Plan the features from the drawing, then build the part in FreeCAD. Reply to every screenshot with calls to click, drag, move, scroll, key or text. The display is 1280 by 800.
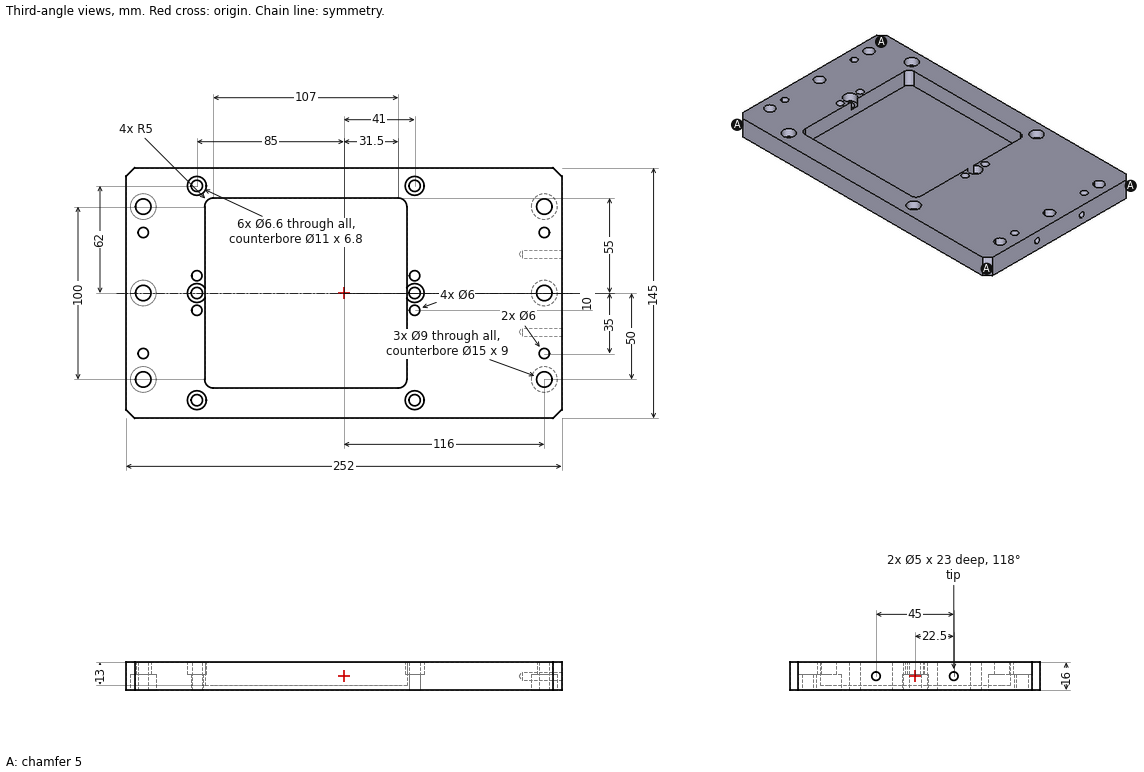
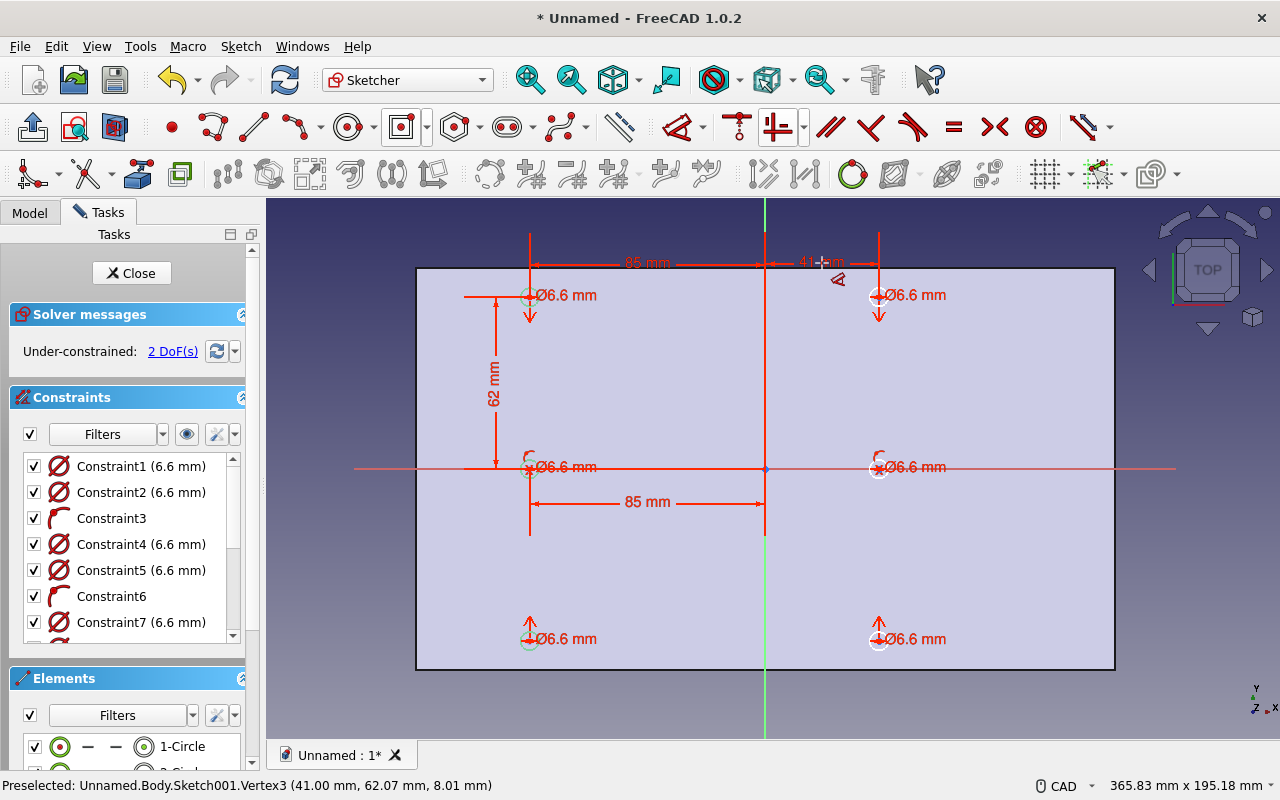
click(879, 297)
click(913, 383)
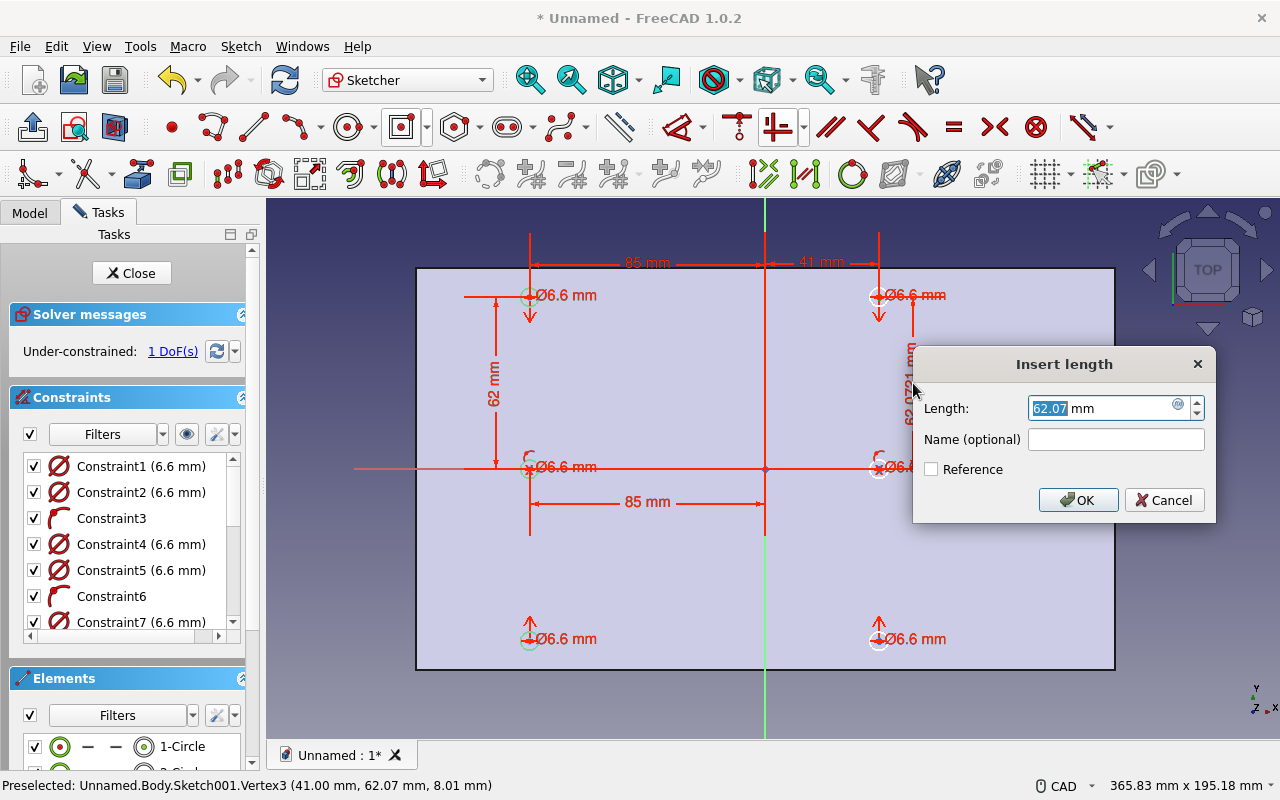
text(62)
key(Return)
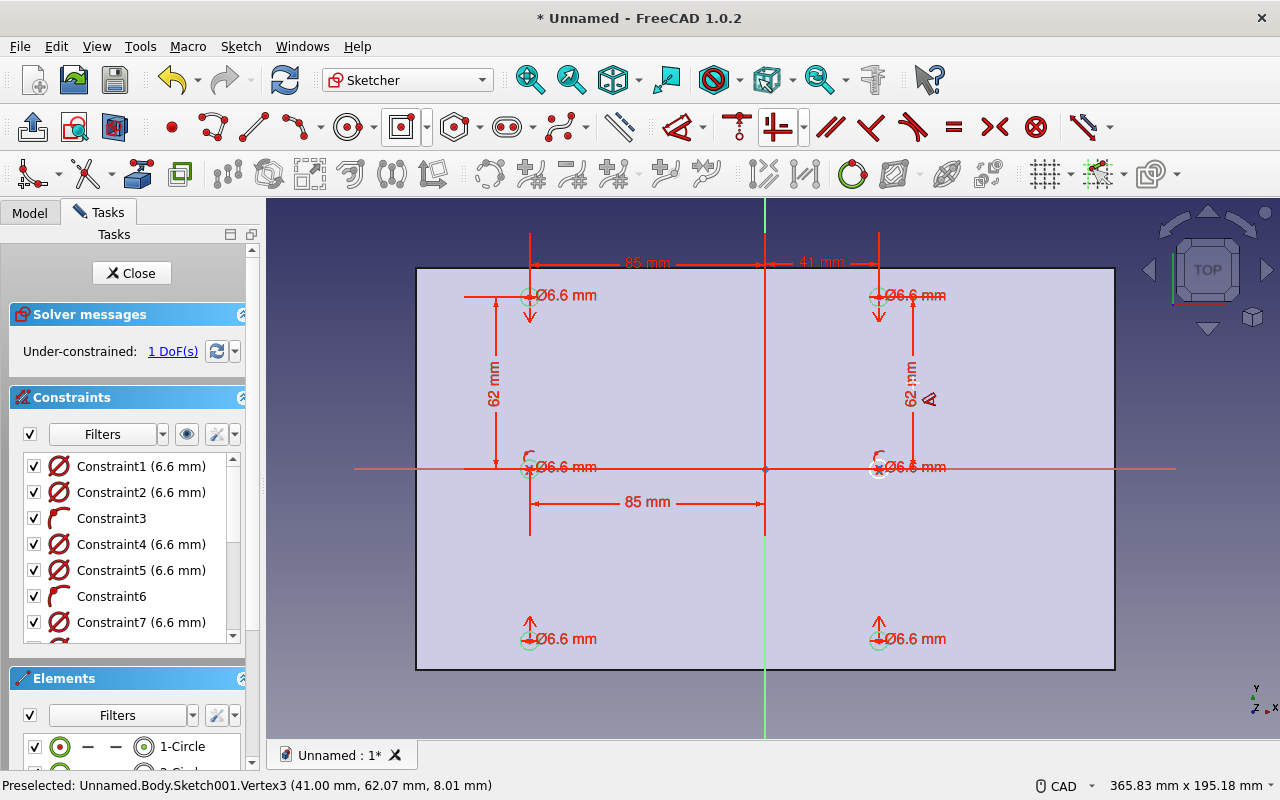
click(879, 469)
click(822, 503)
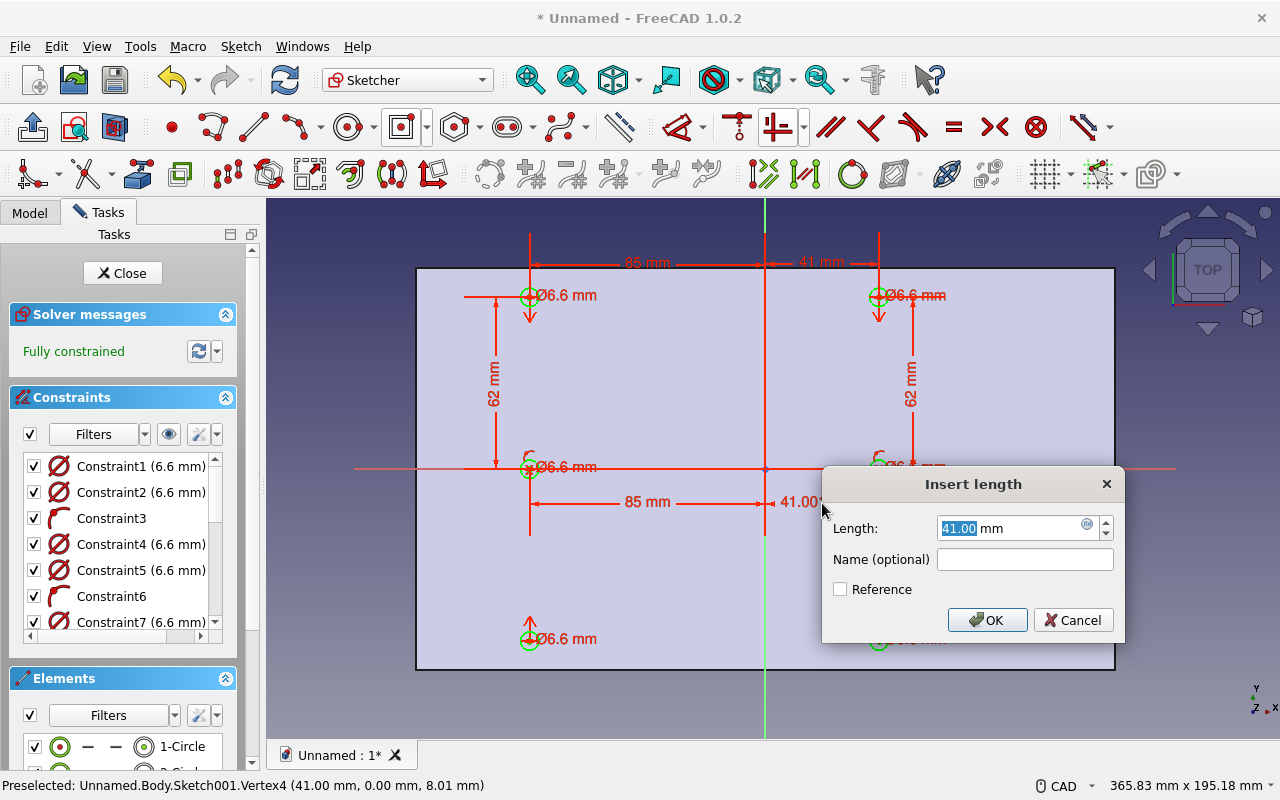
text(41)
key(Return)
key(Escape)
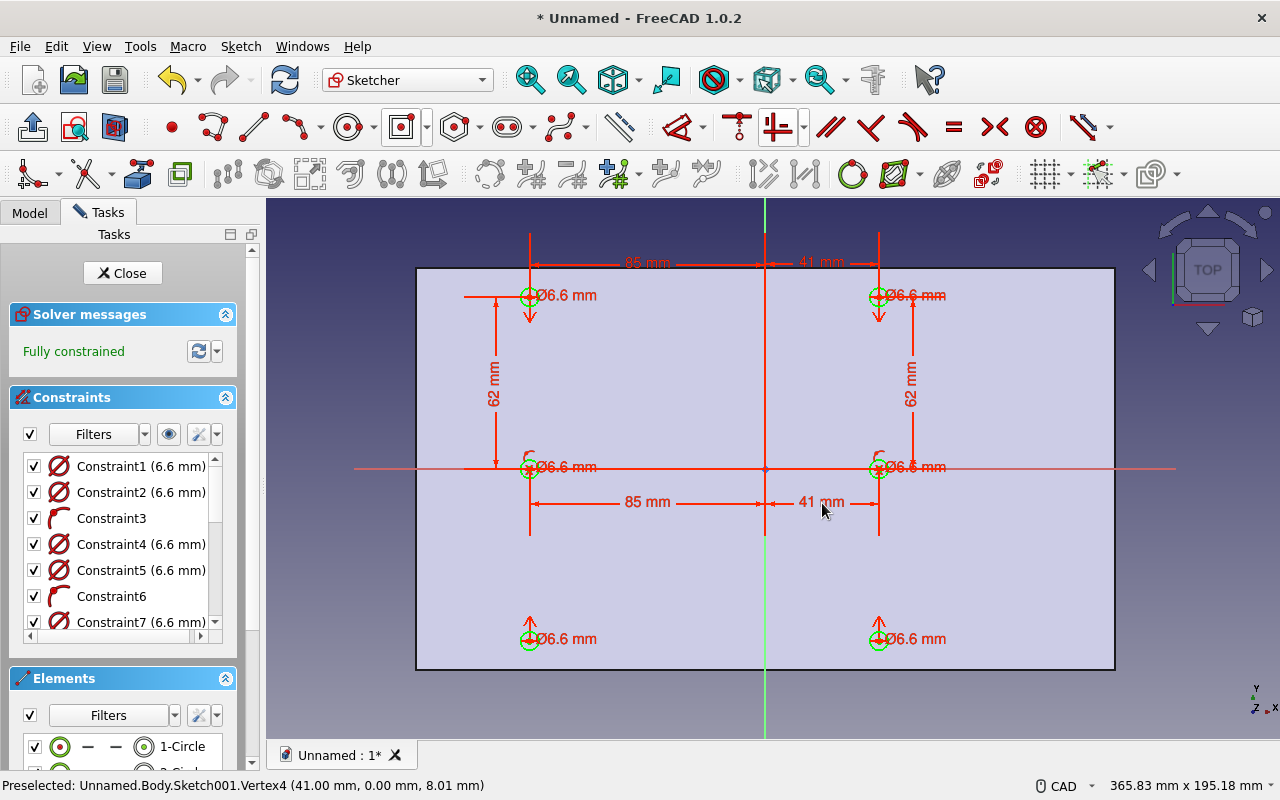
click(123, 273)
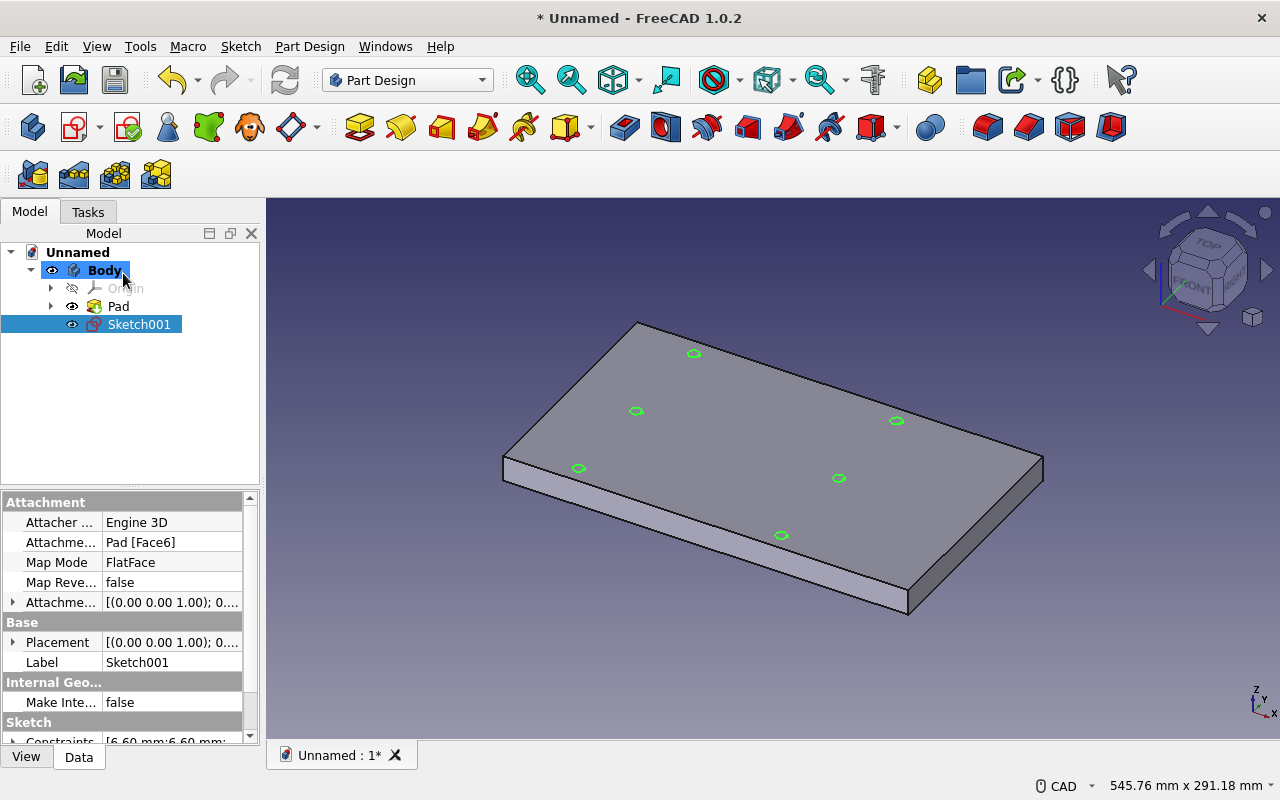
click(666, 128)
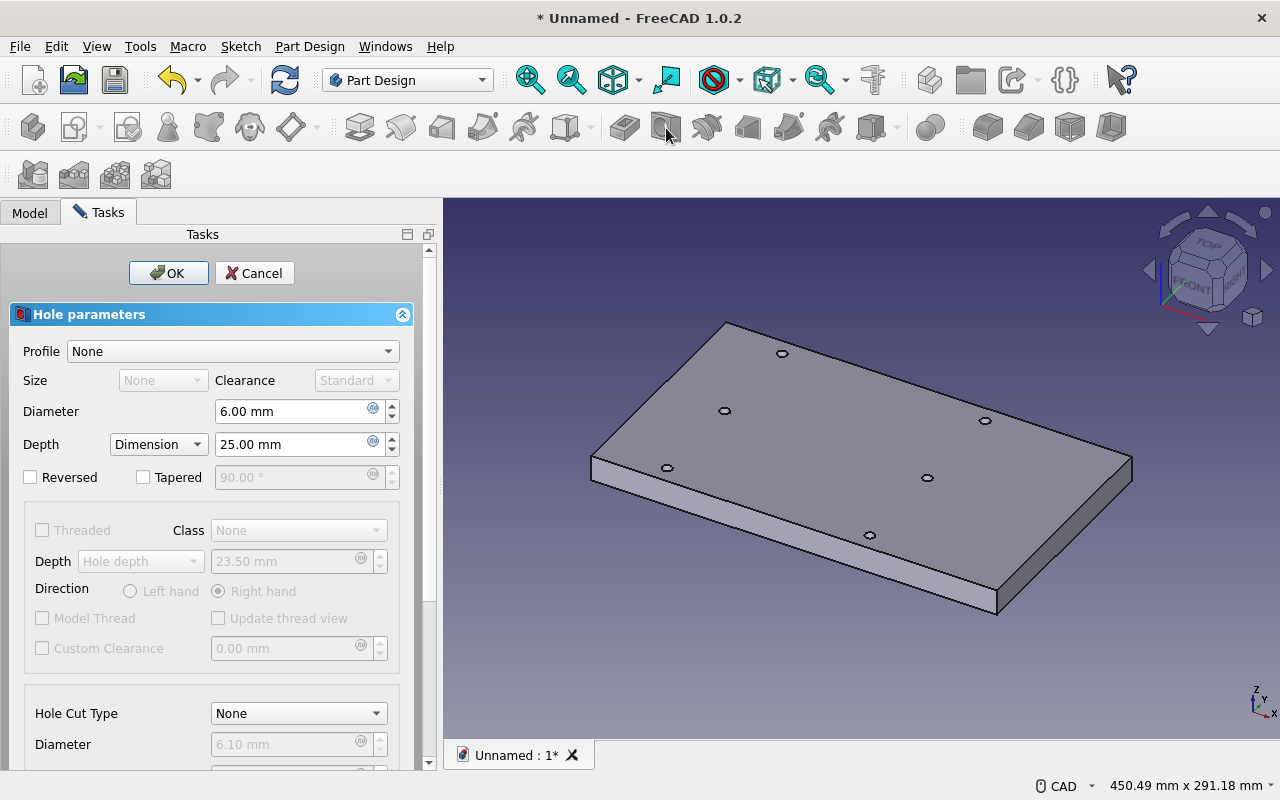
triple_click(300, 412)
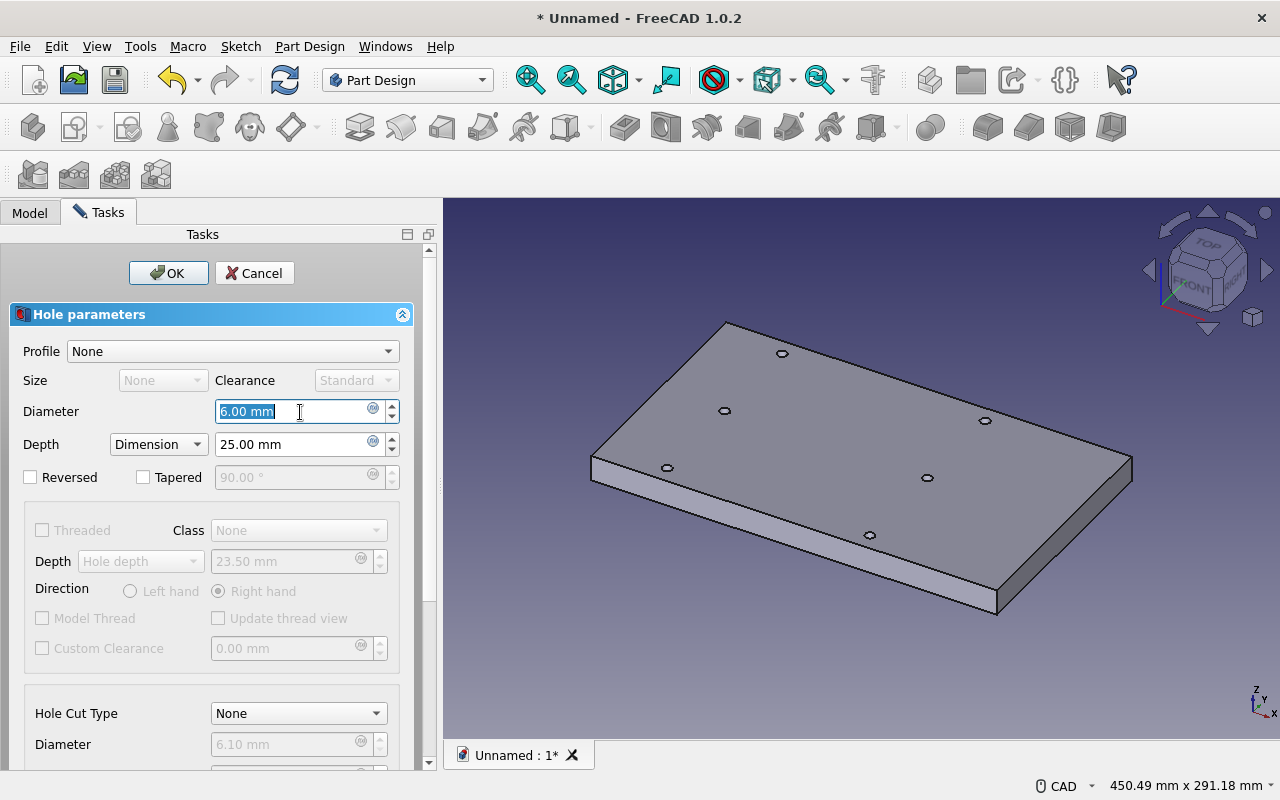
text(6.6)
key(Tab)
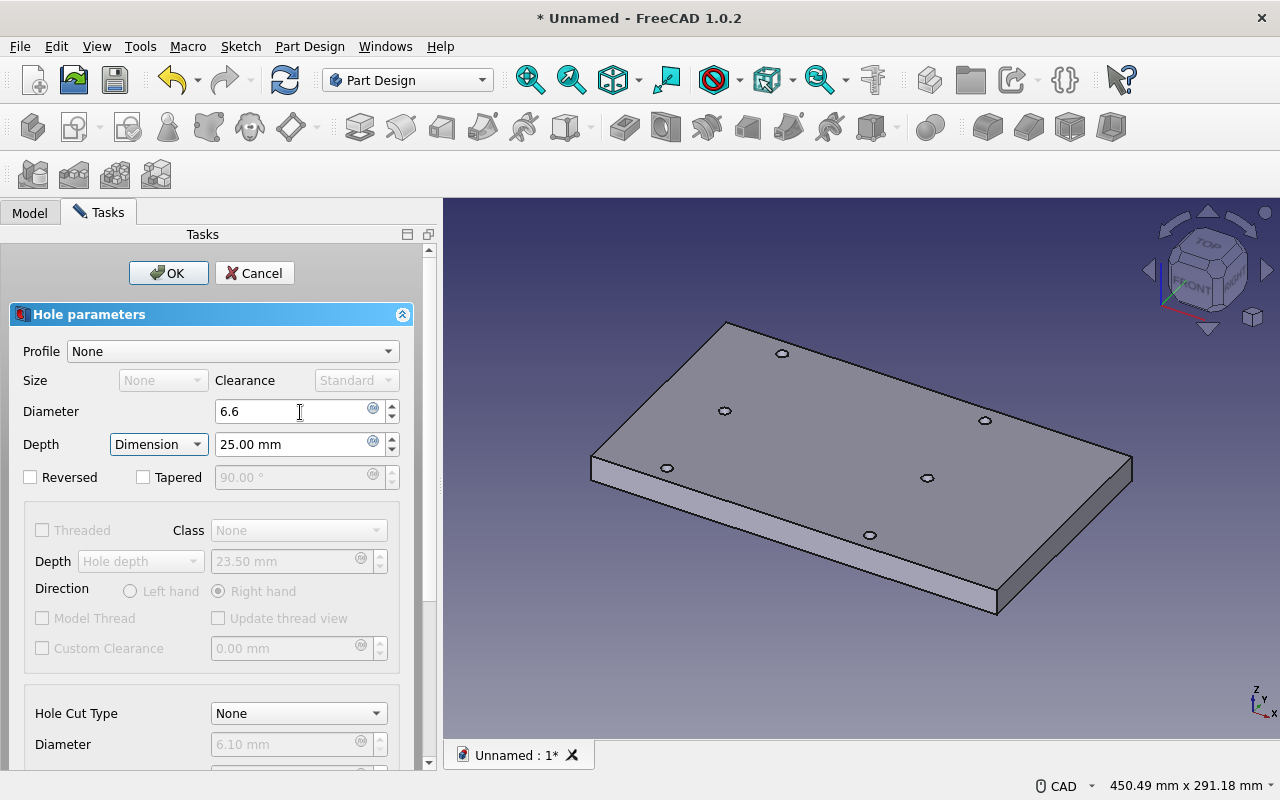
click(160, 444)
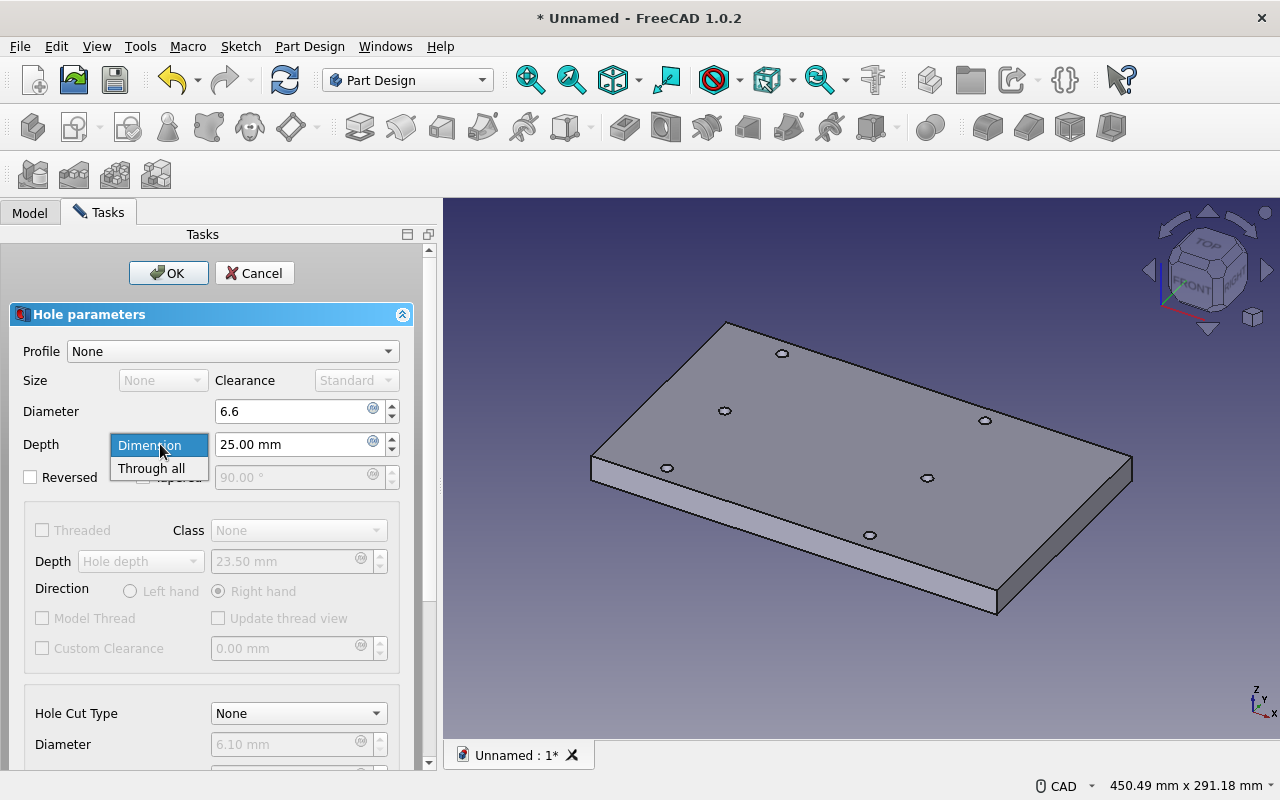
click(158, 468)